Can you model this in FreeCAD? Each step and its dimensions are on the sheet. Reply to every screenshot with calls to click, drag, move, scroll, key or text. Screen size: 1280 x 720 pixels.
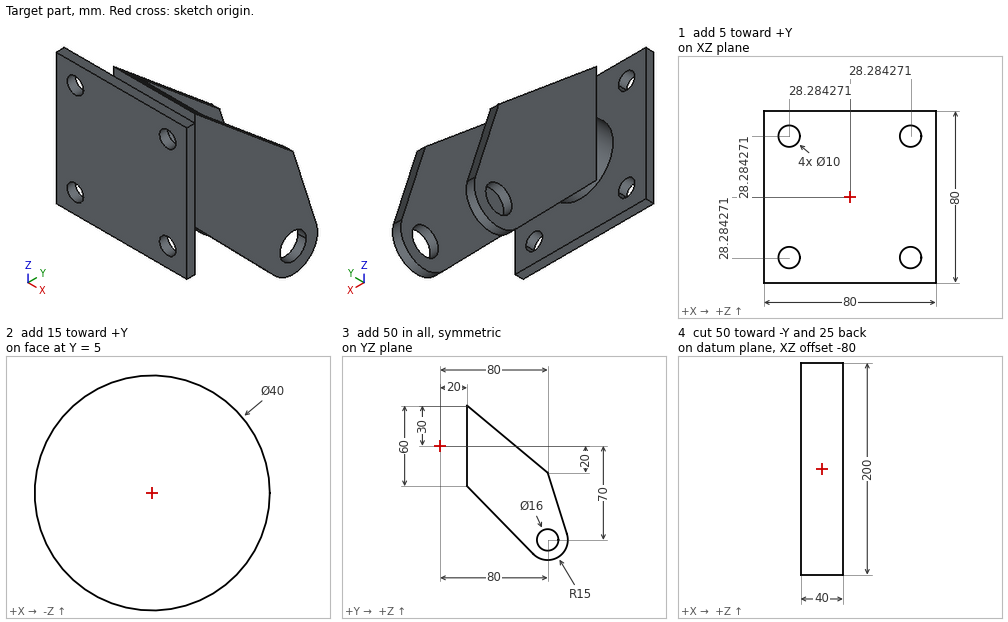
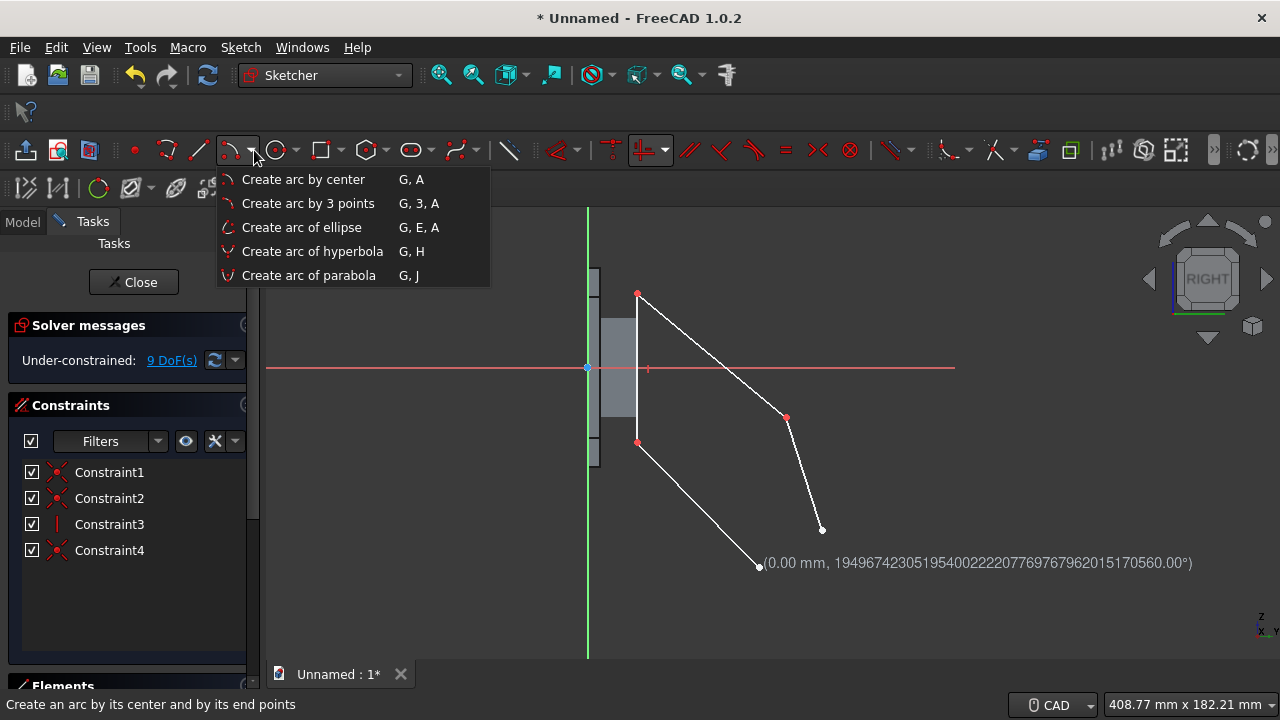
click(354, 203)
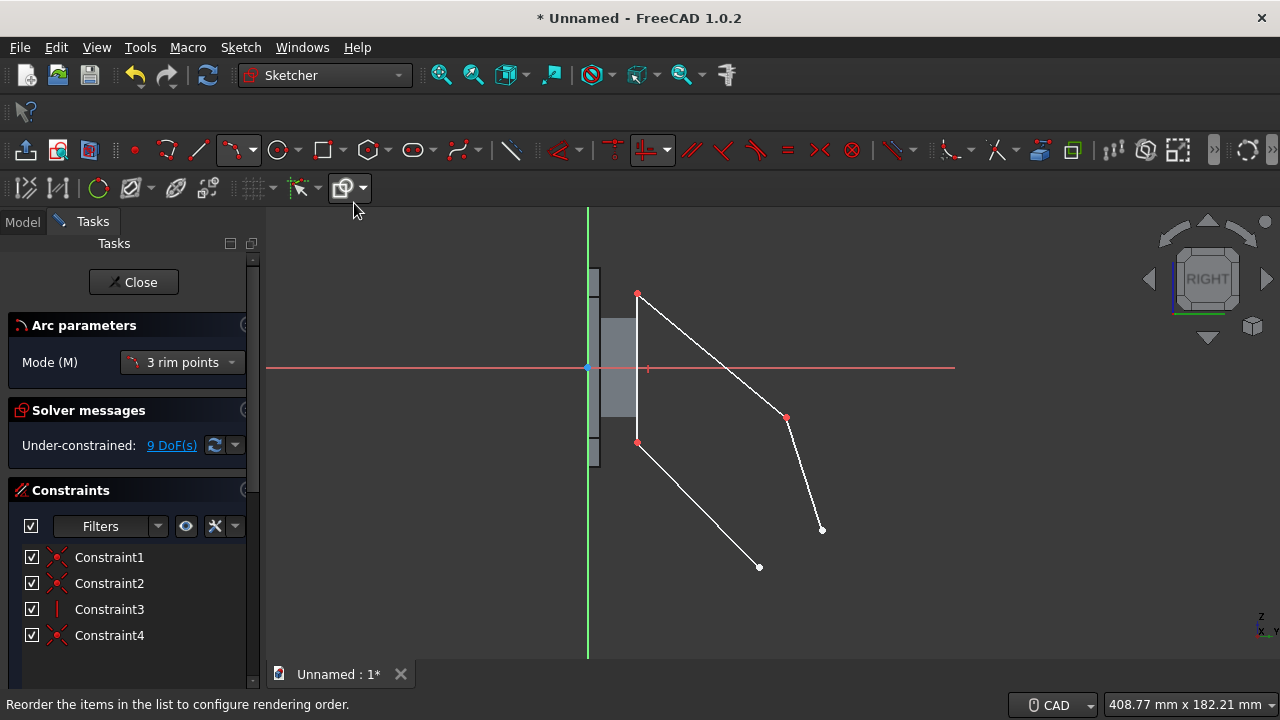
click(759, 568)
click(822, 531)
click(805, 573)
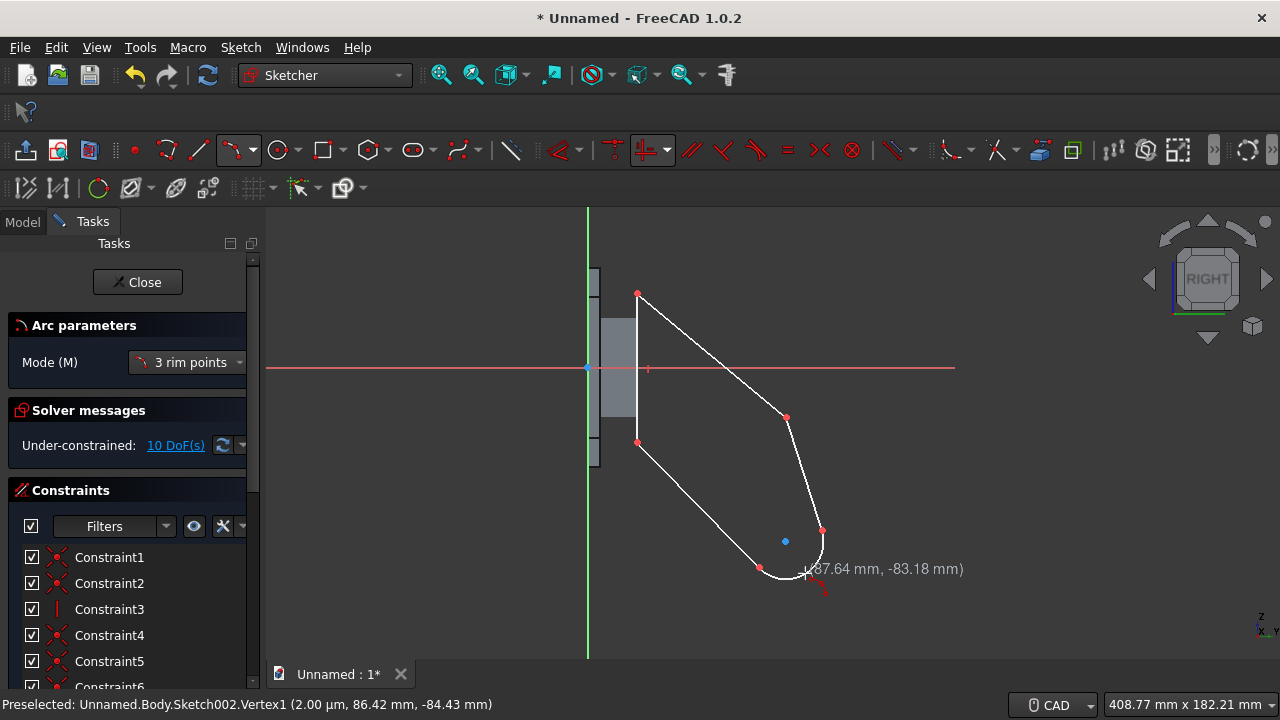
click(278, 150)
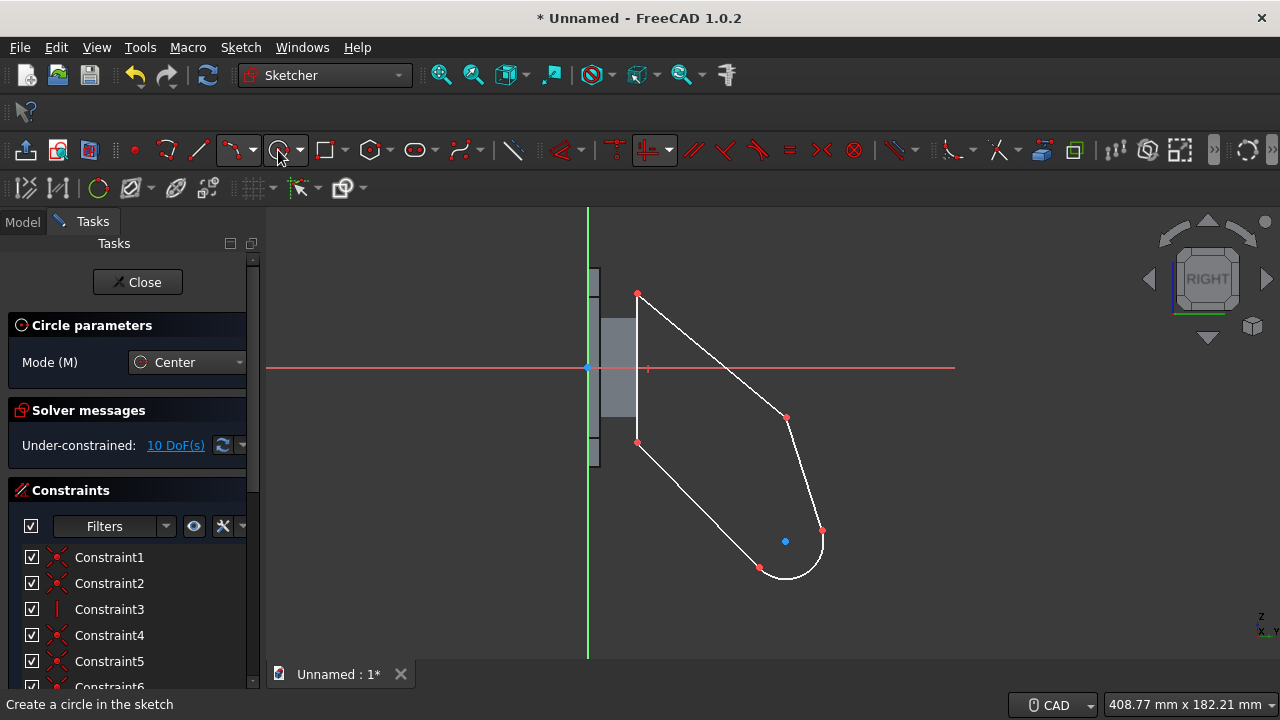
click(786, 541)
click(800, 527)
key(Escape)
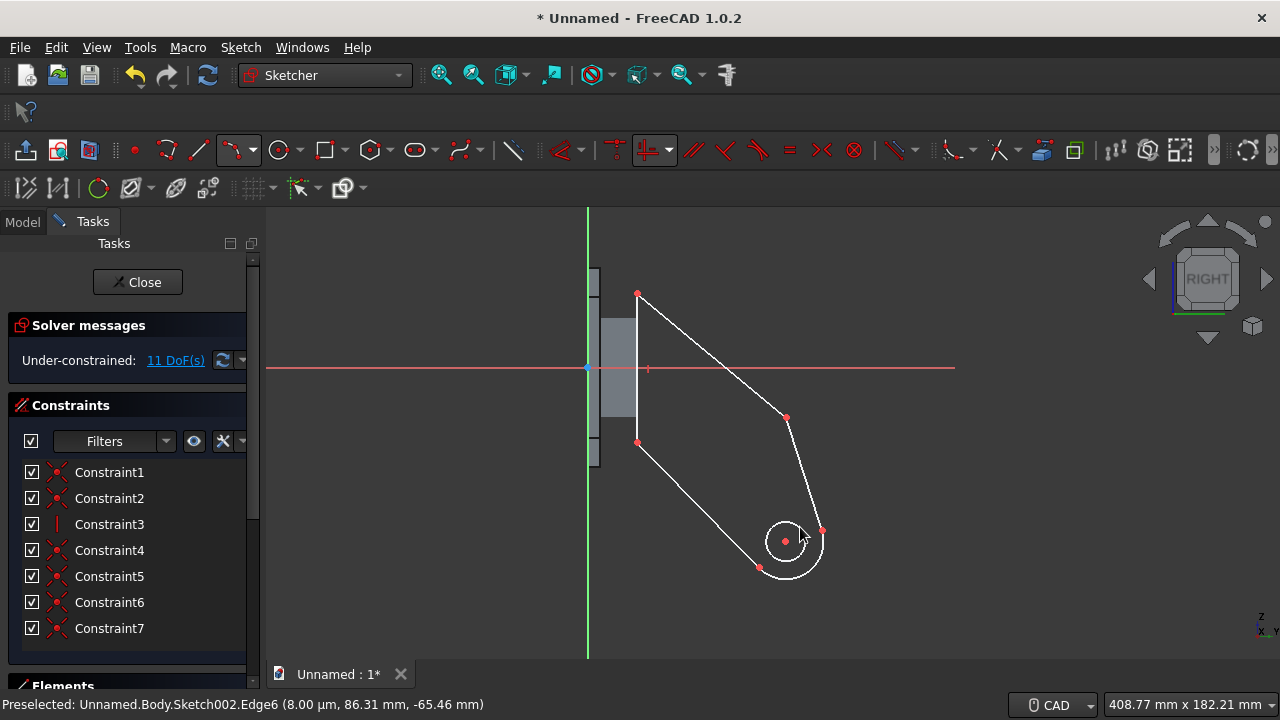
click(811, 497)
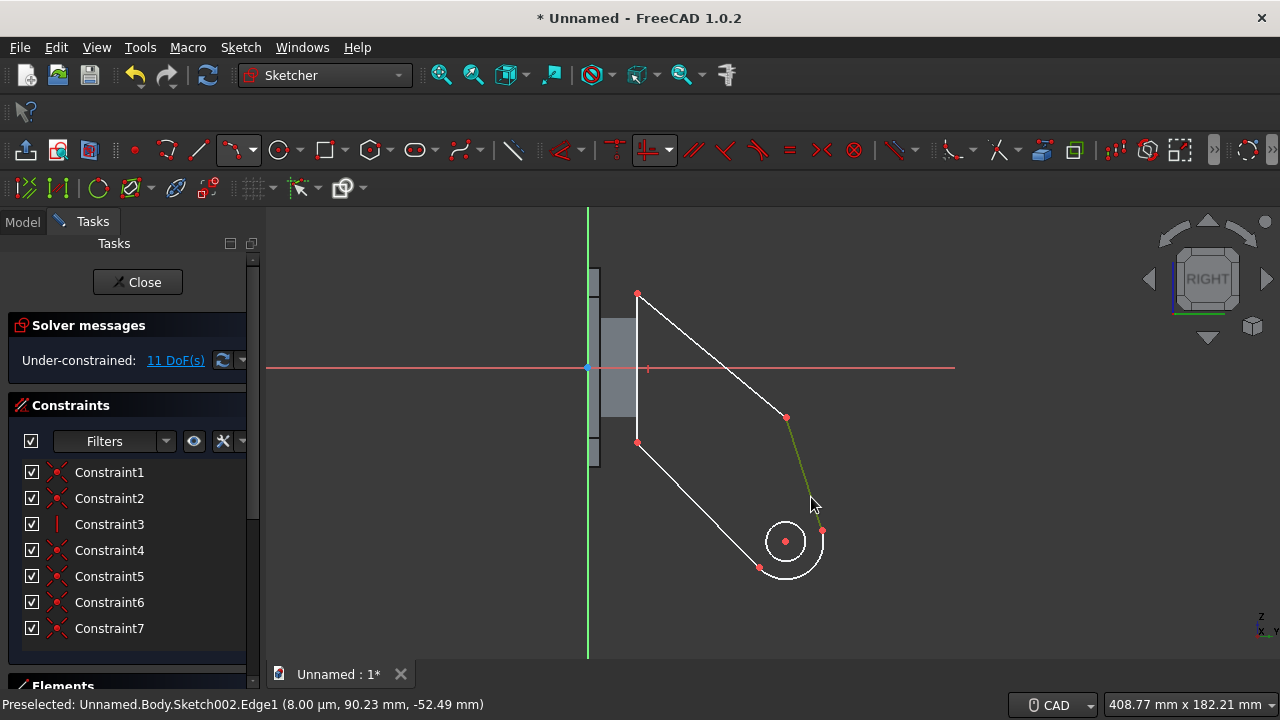
click(786, 579)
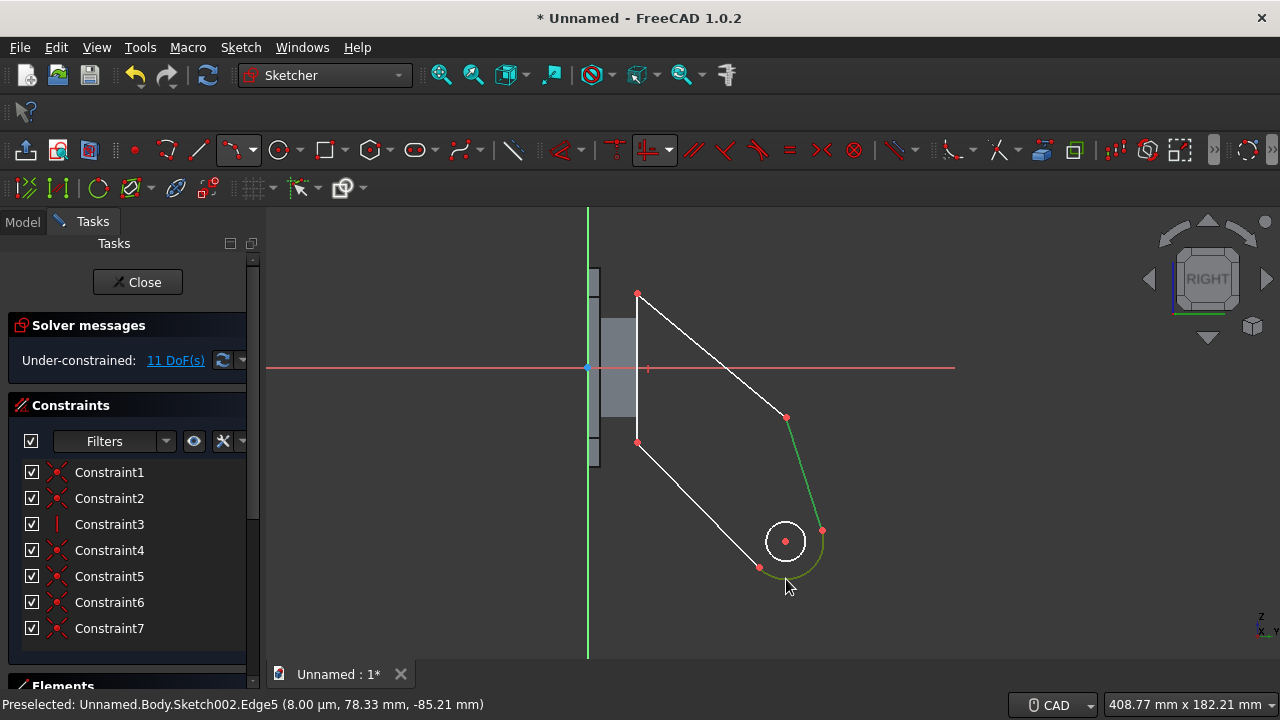
click(758, 150)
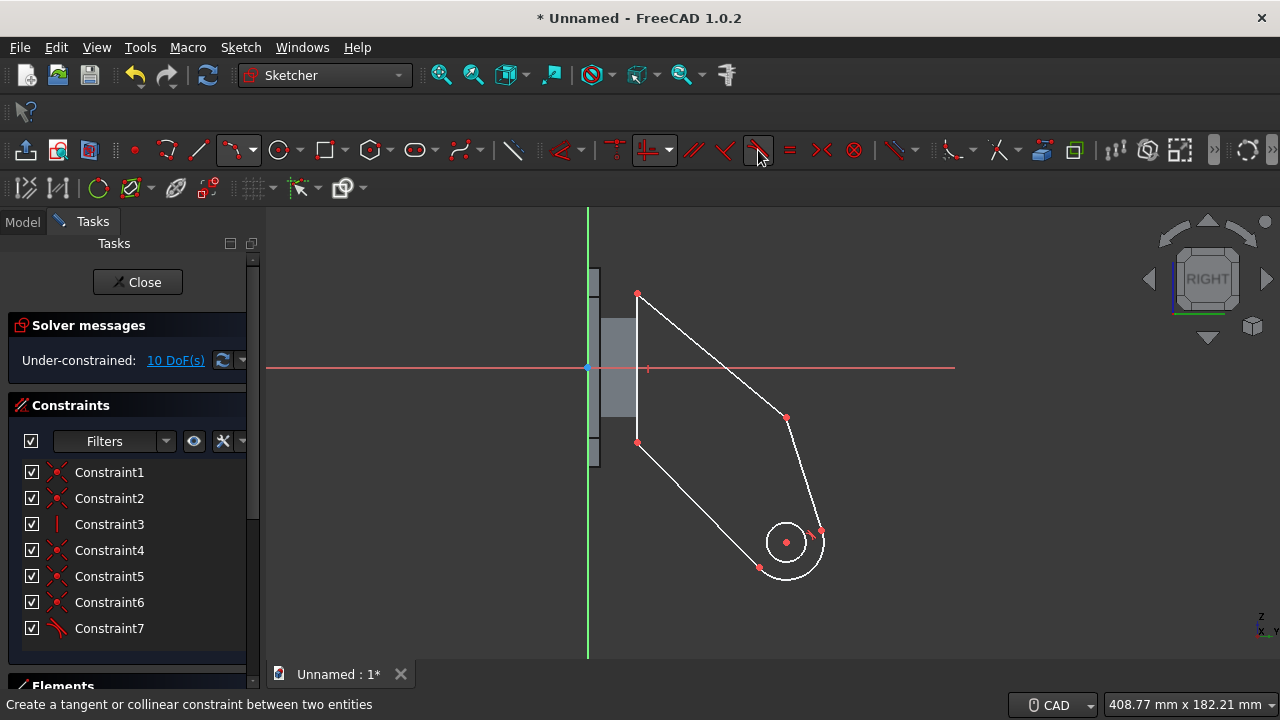
click(674, 481)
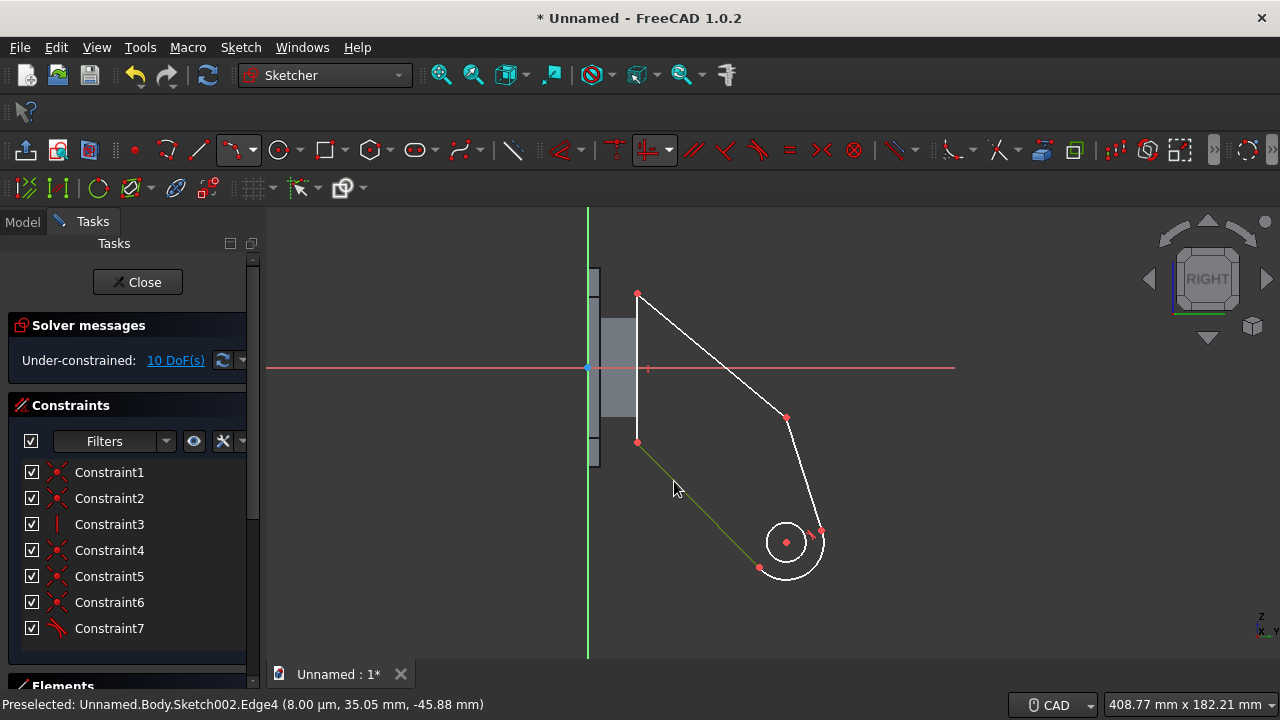
click(786, 580)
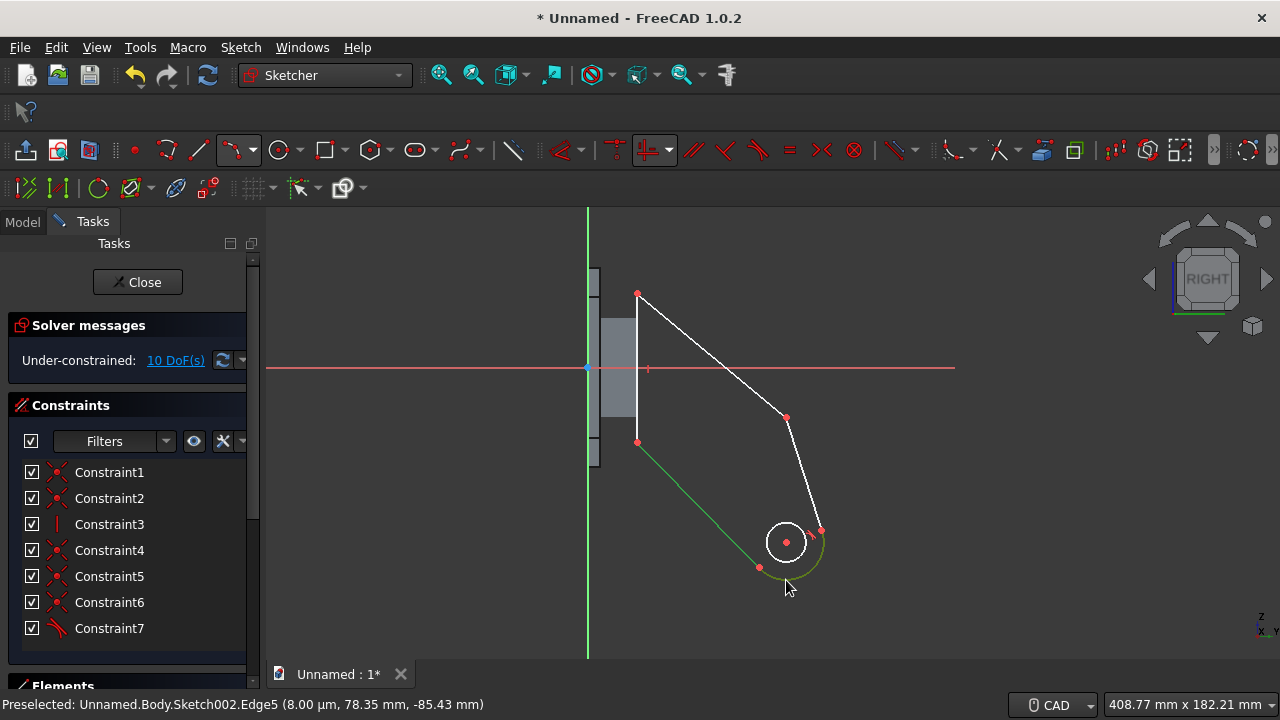
click(758, 150)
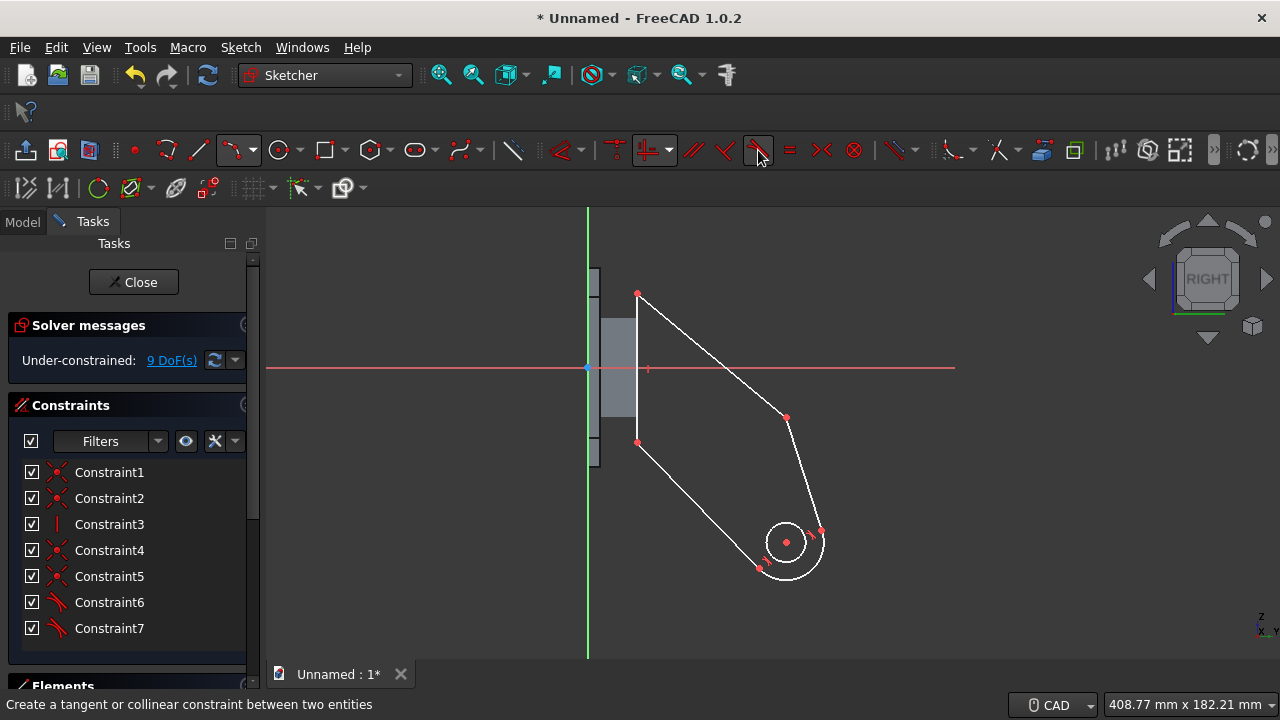
click(560, 150)